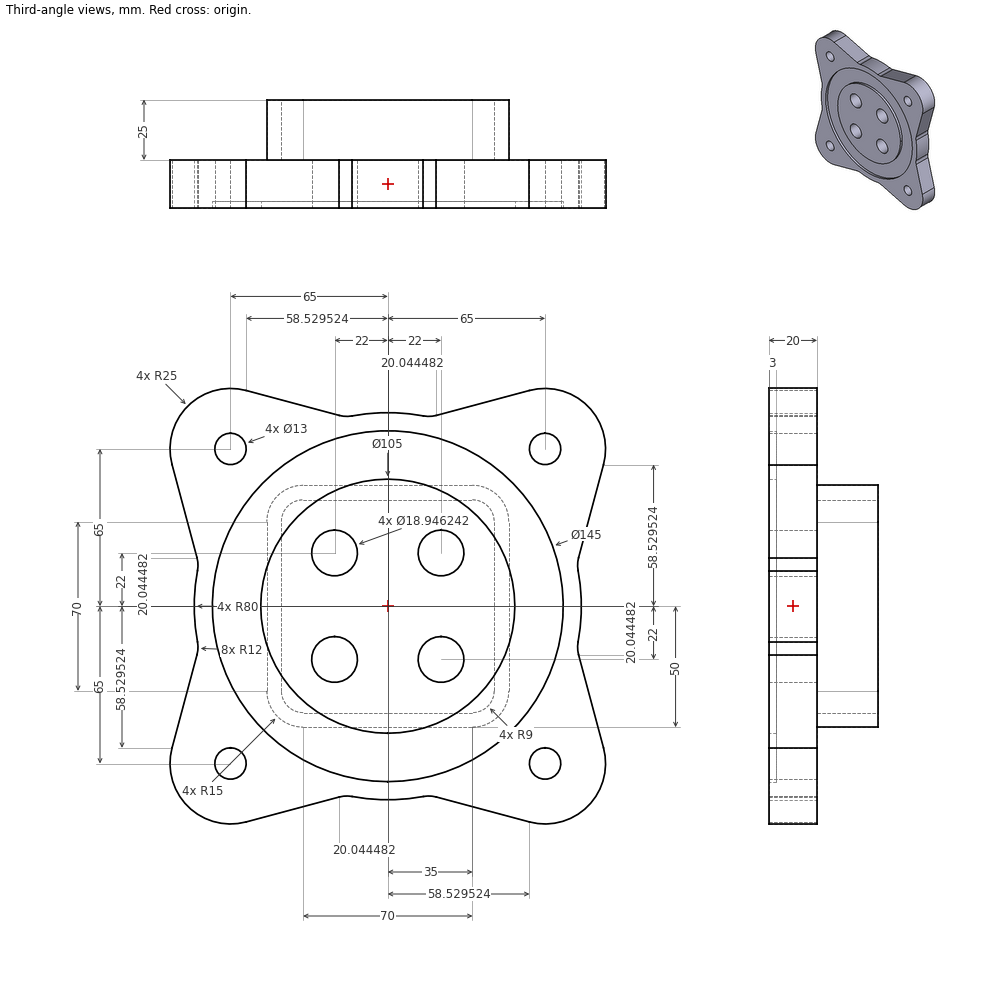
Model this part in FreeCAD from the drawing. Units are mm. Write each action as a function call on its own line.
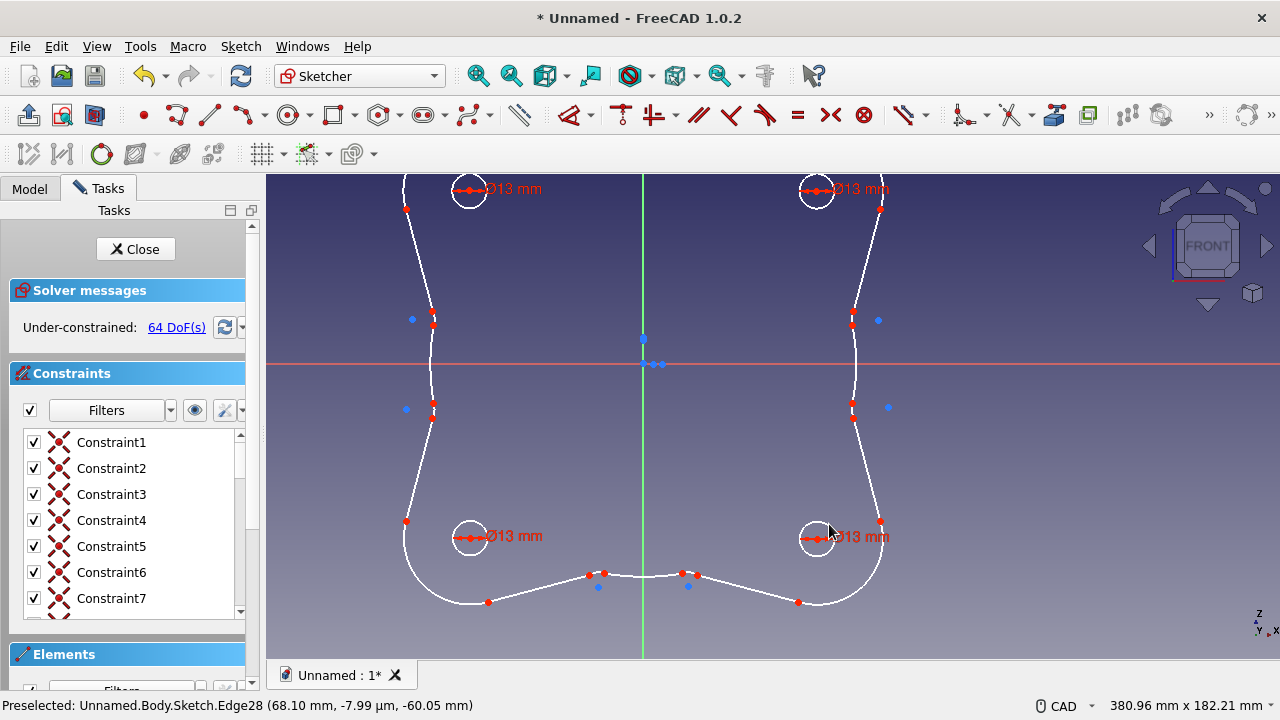
click(414, 491)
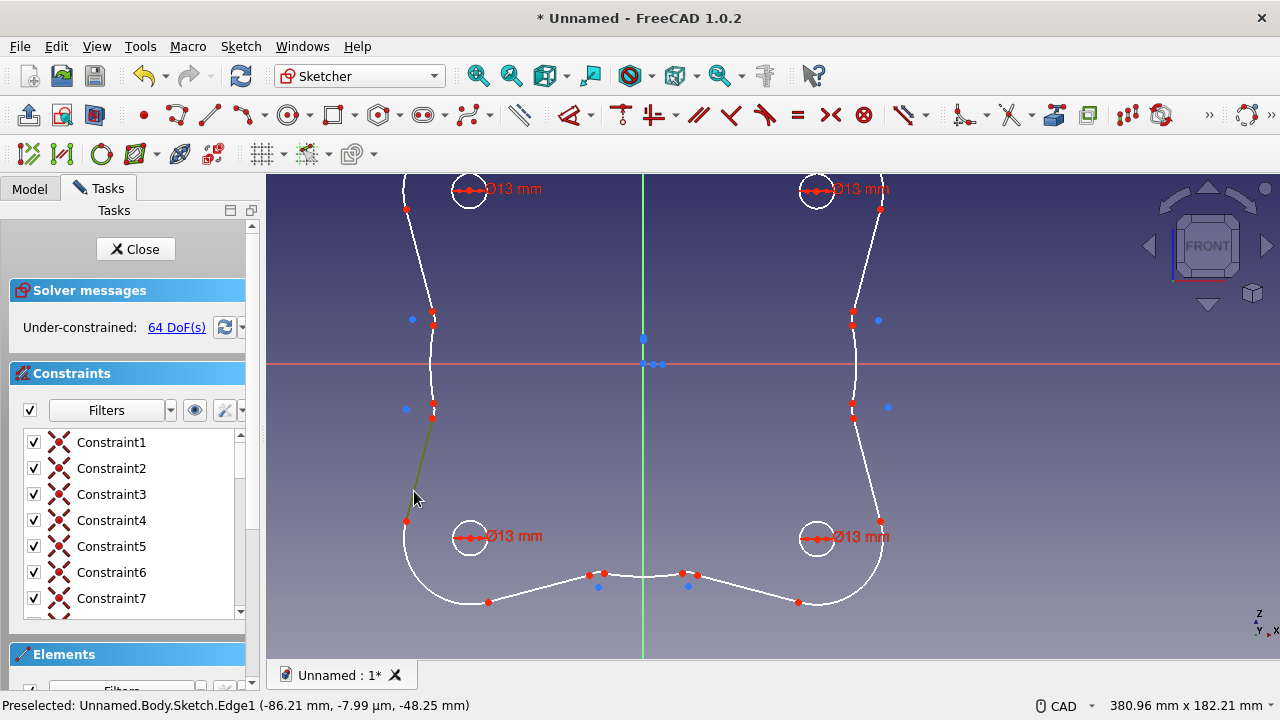
scroll(434, 411, up, 3)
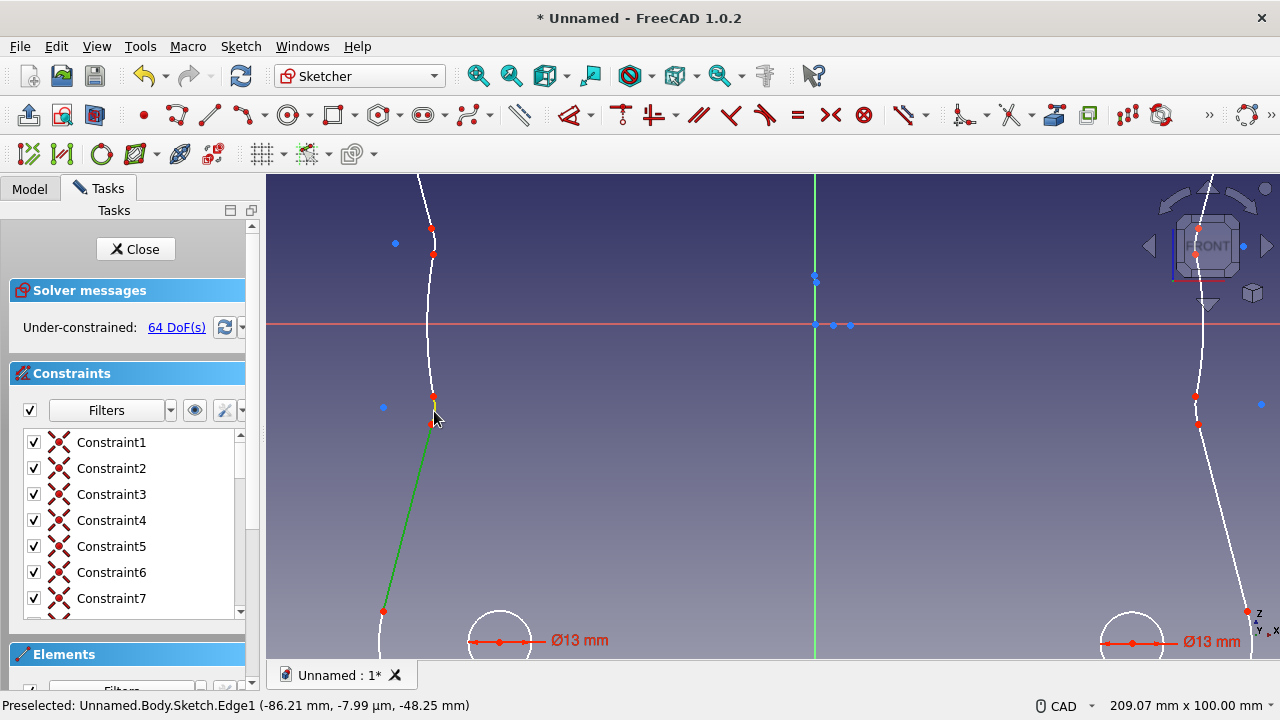
click(435, 411)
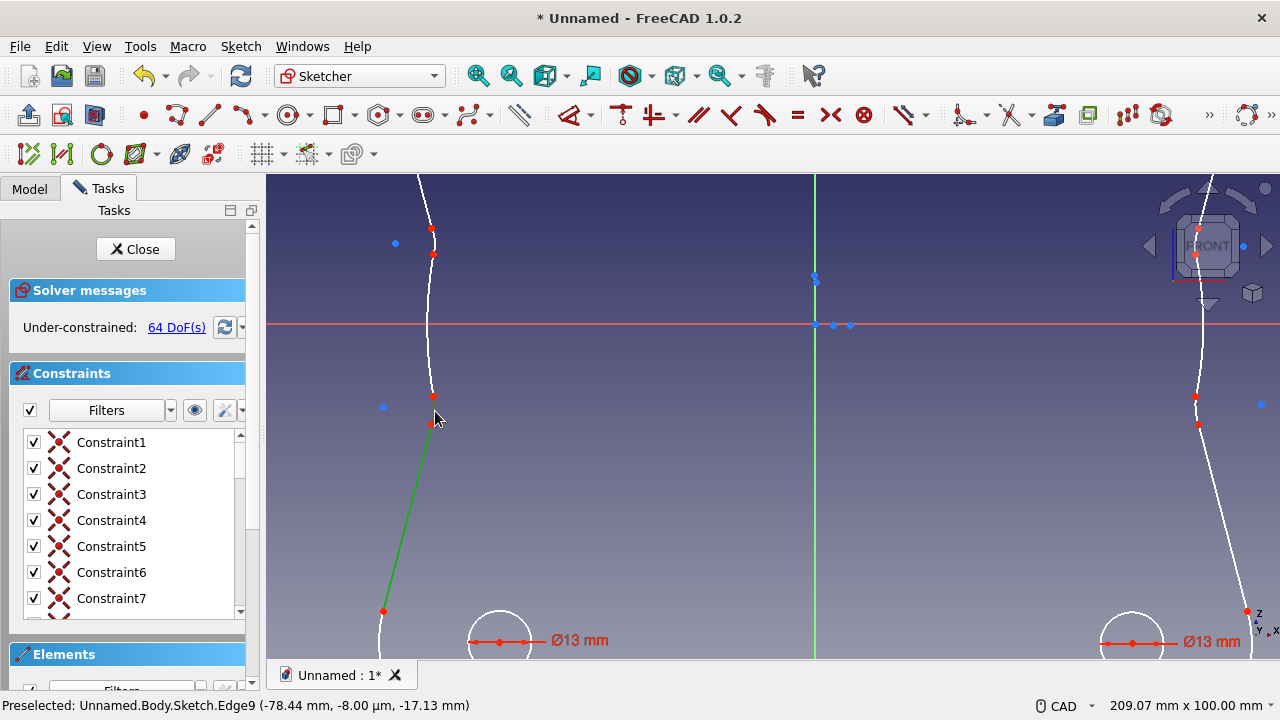
click(765, 116)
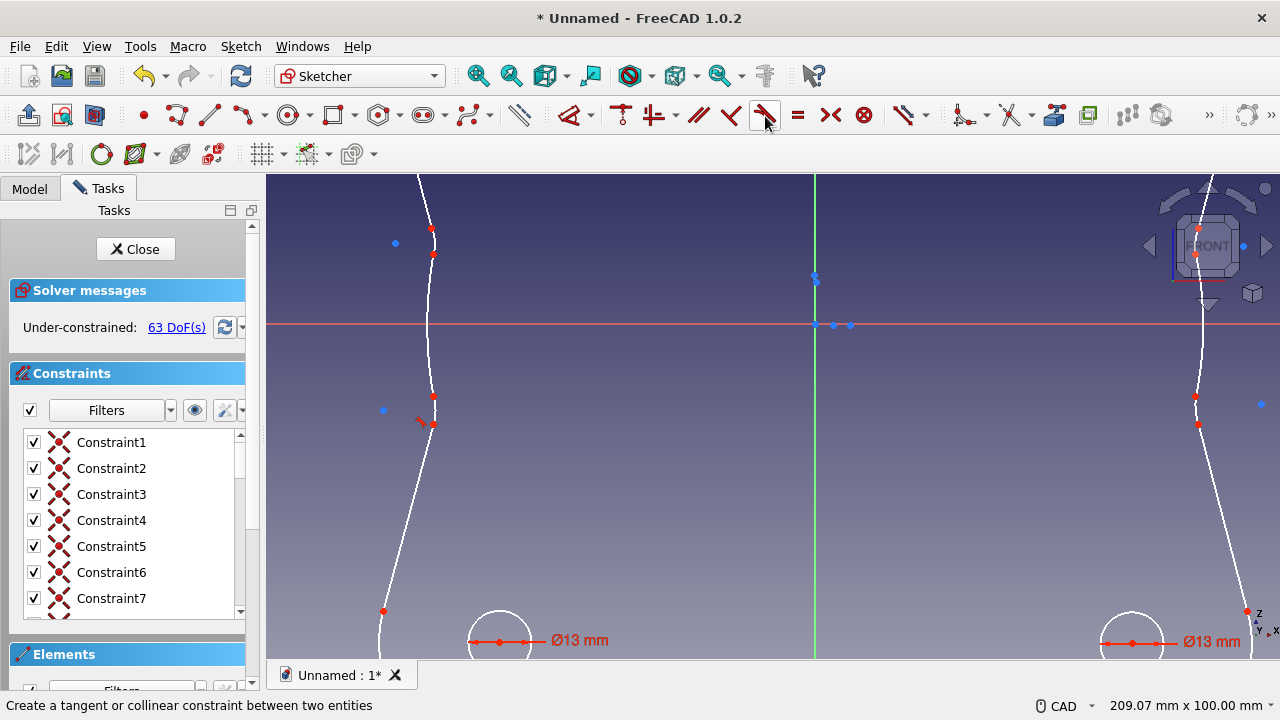
click(398, 556)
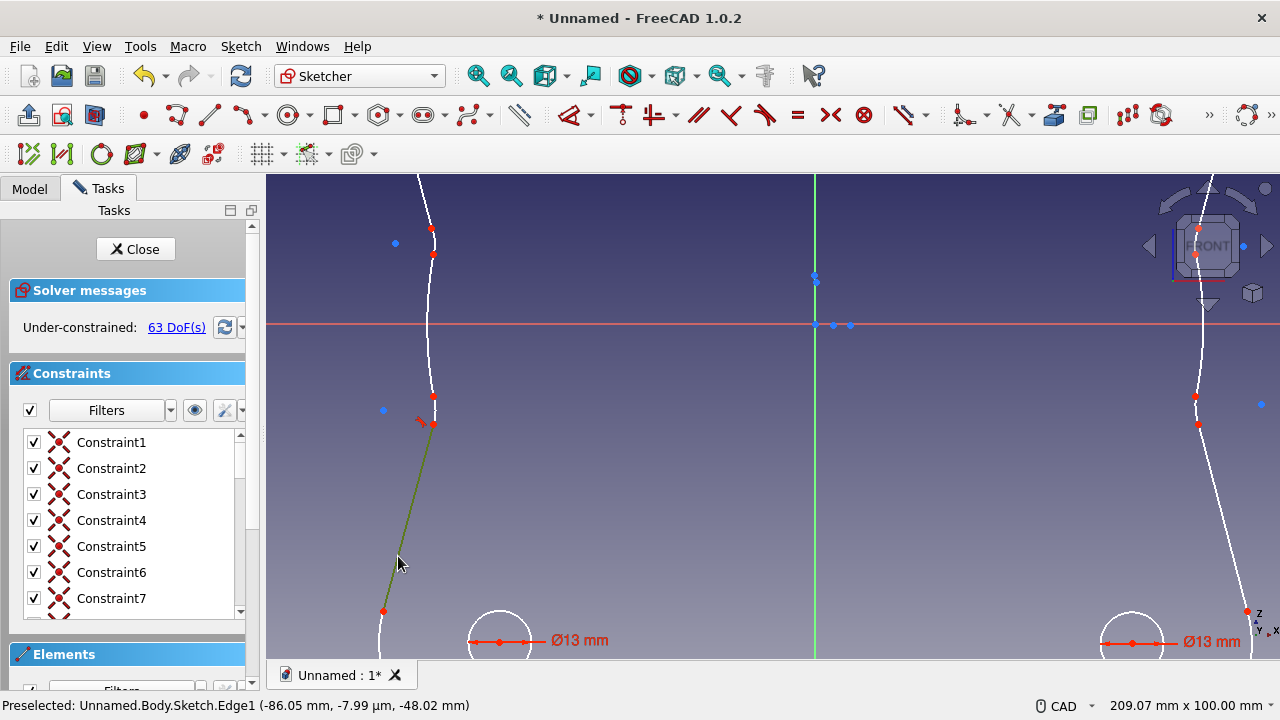
scroll(640, 470, down, 5)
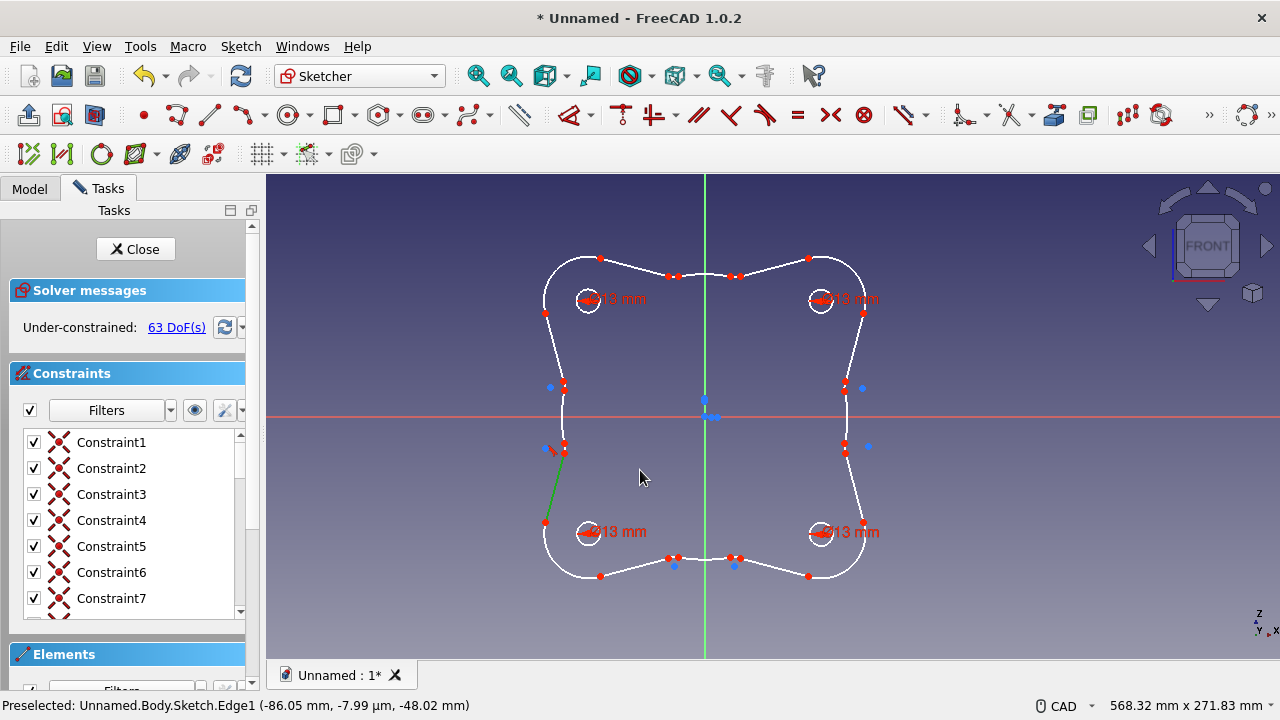
click(547, 550)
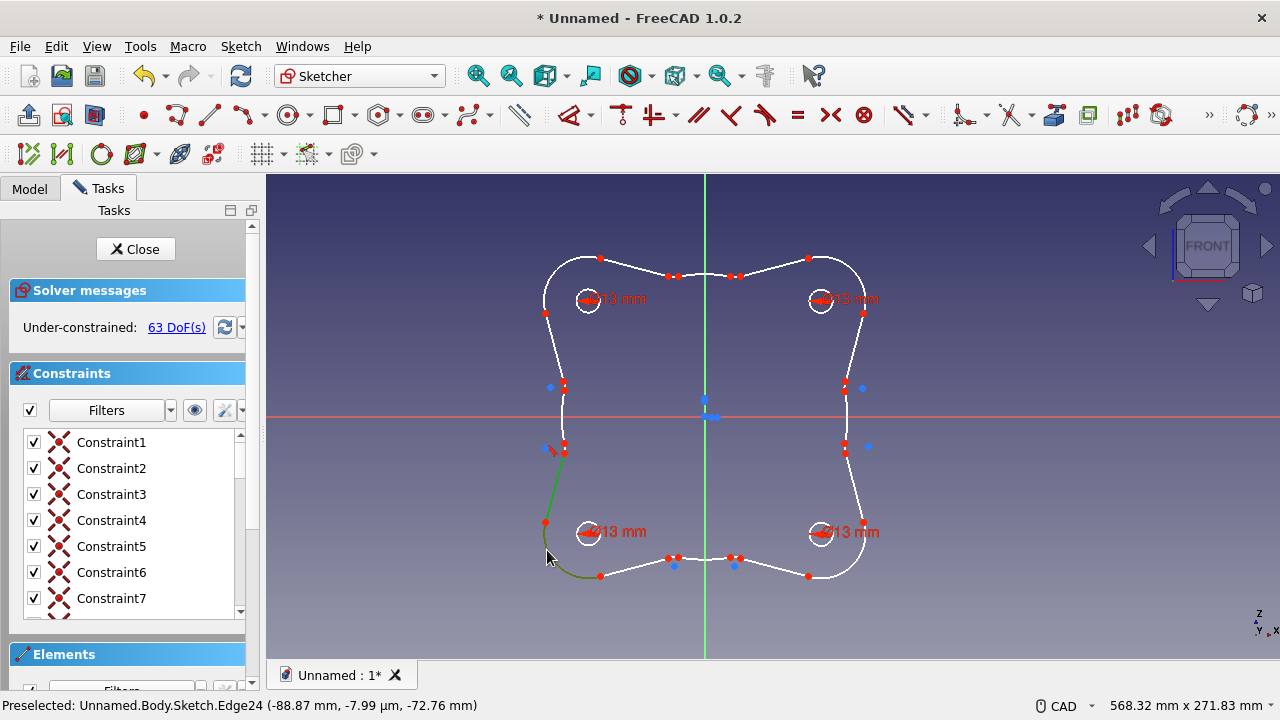
click(765, 116)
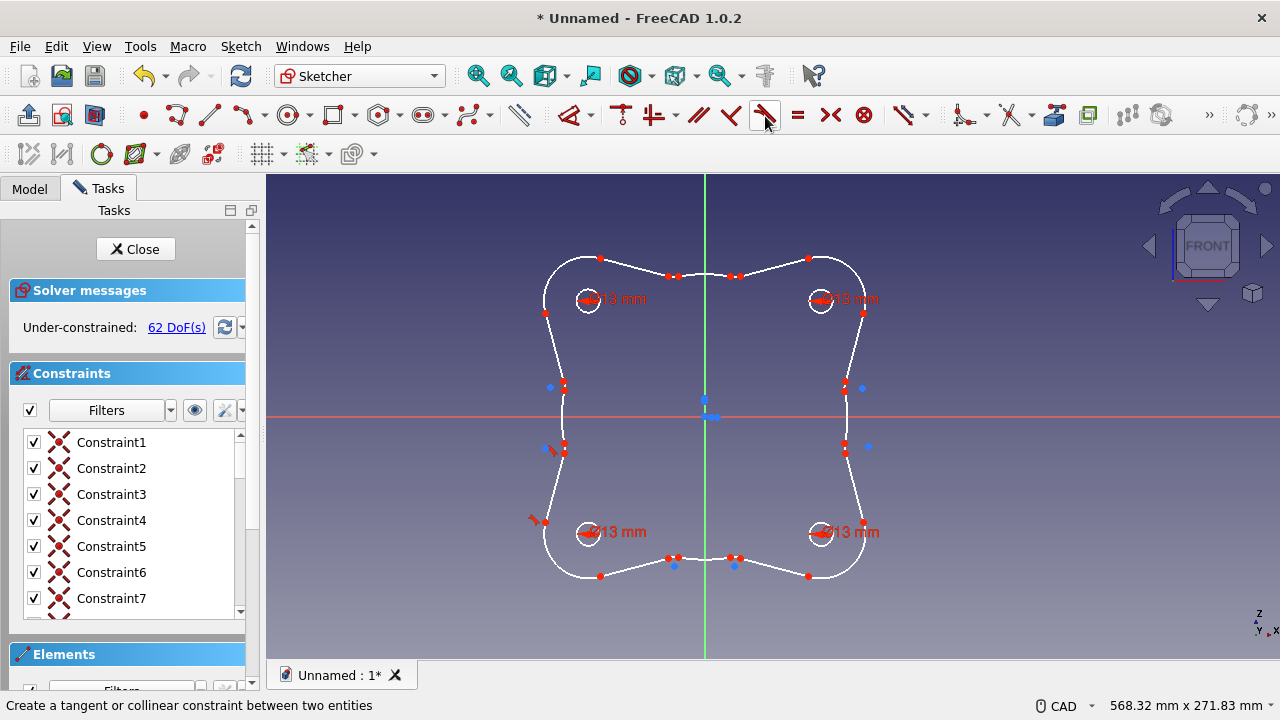
click(558, 361)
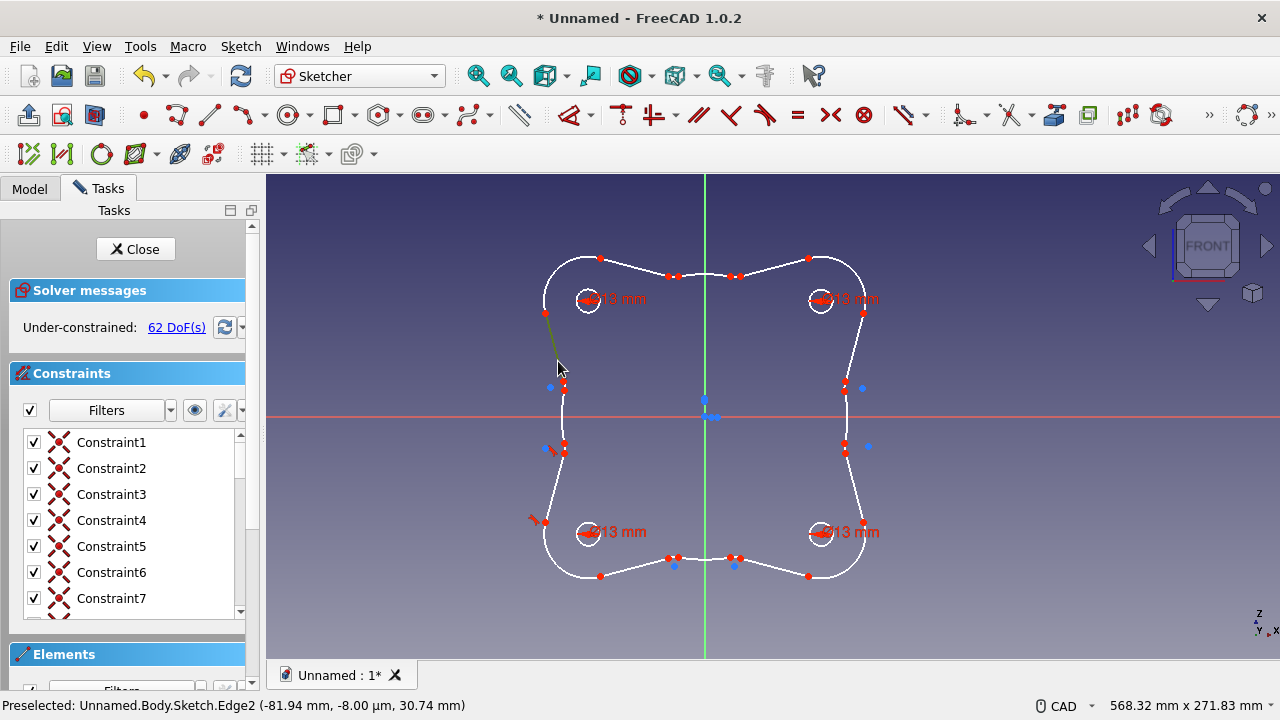
scroll(565, 386, up, 6)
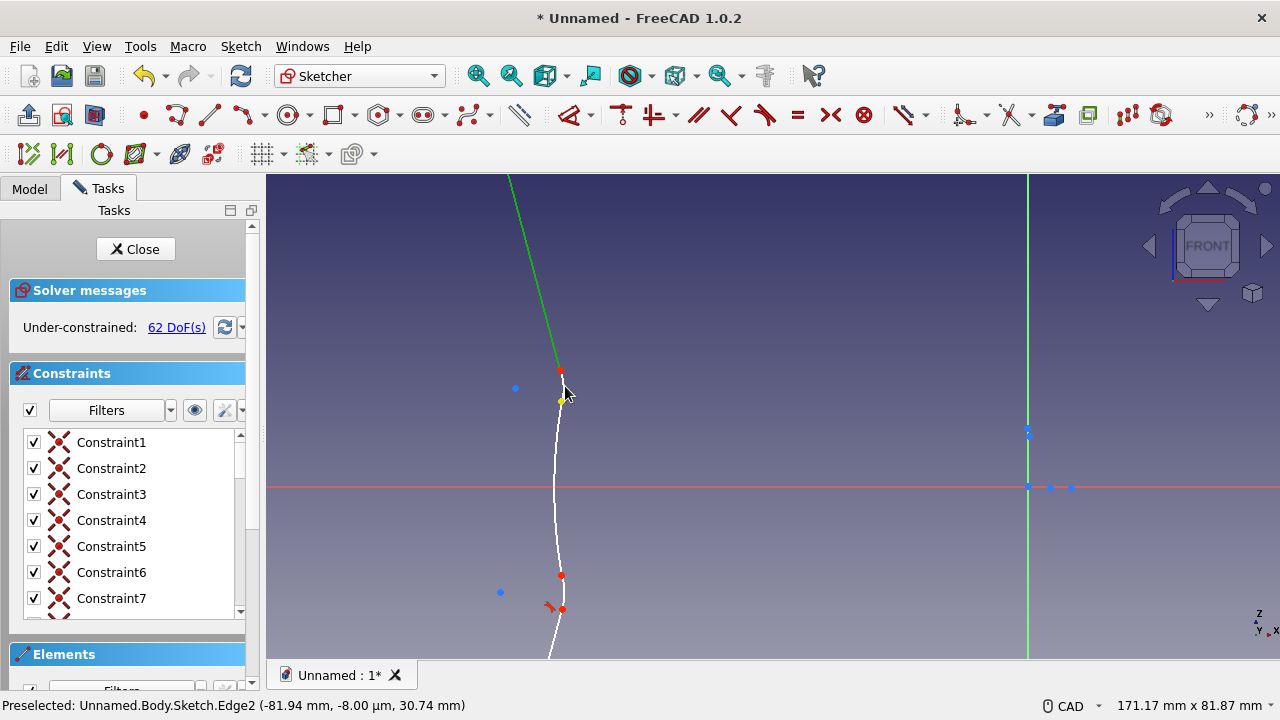
click(564, 386)